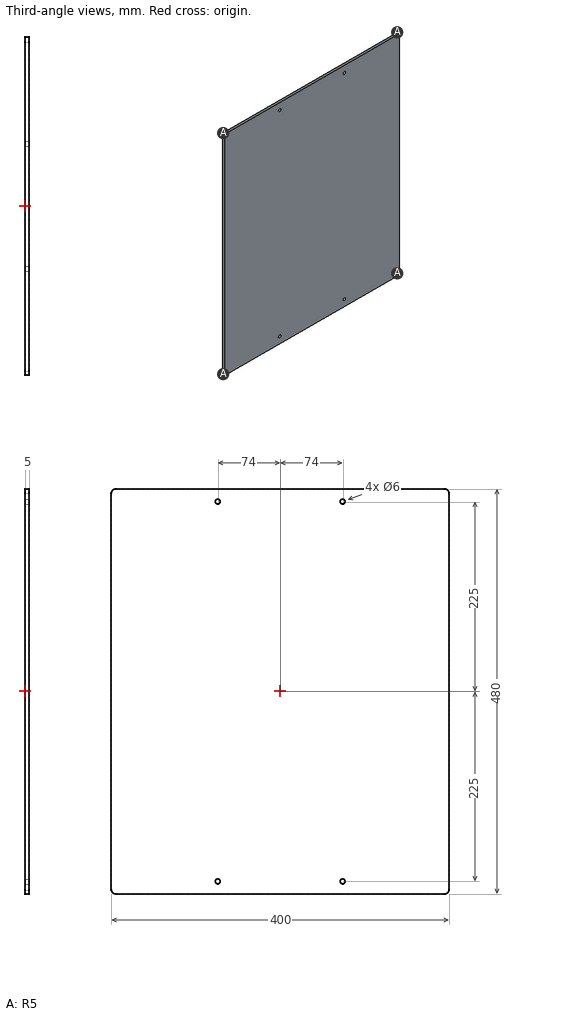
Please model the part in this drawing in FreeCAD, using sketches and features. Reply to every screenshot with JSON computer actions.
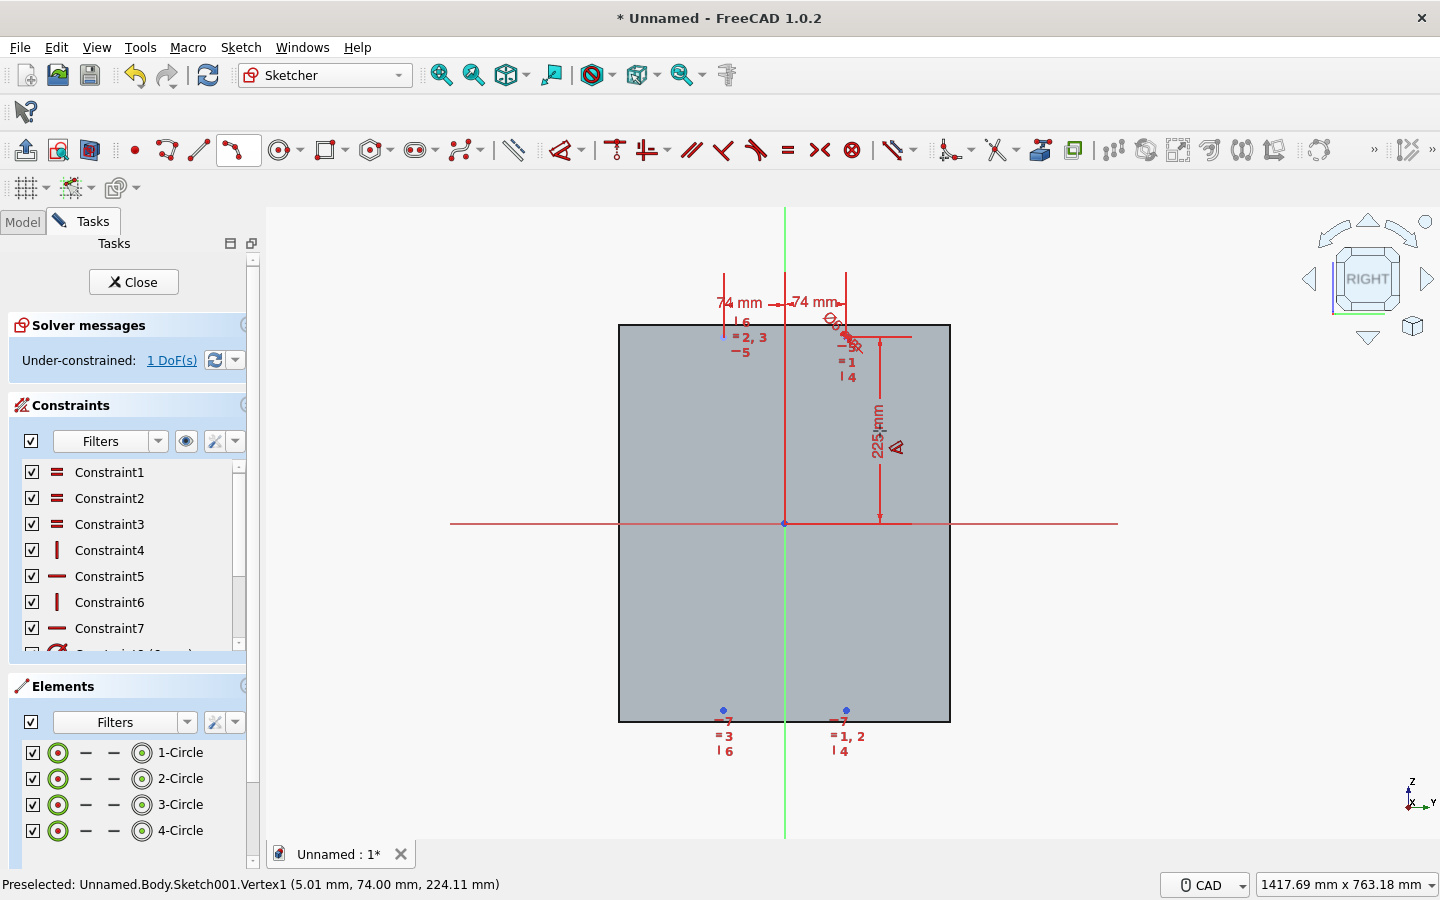
{"action": "left_click", "coordinate": [846, 711]}
{"action": "left_click", "coordinate": [880, 617]}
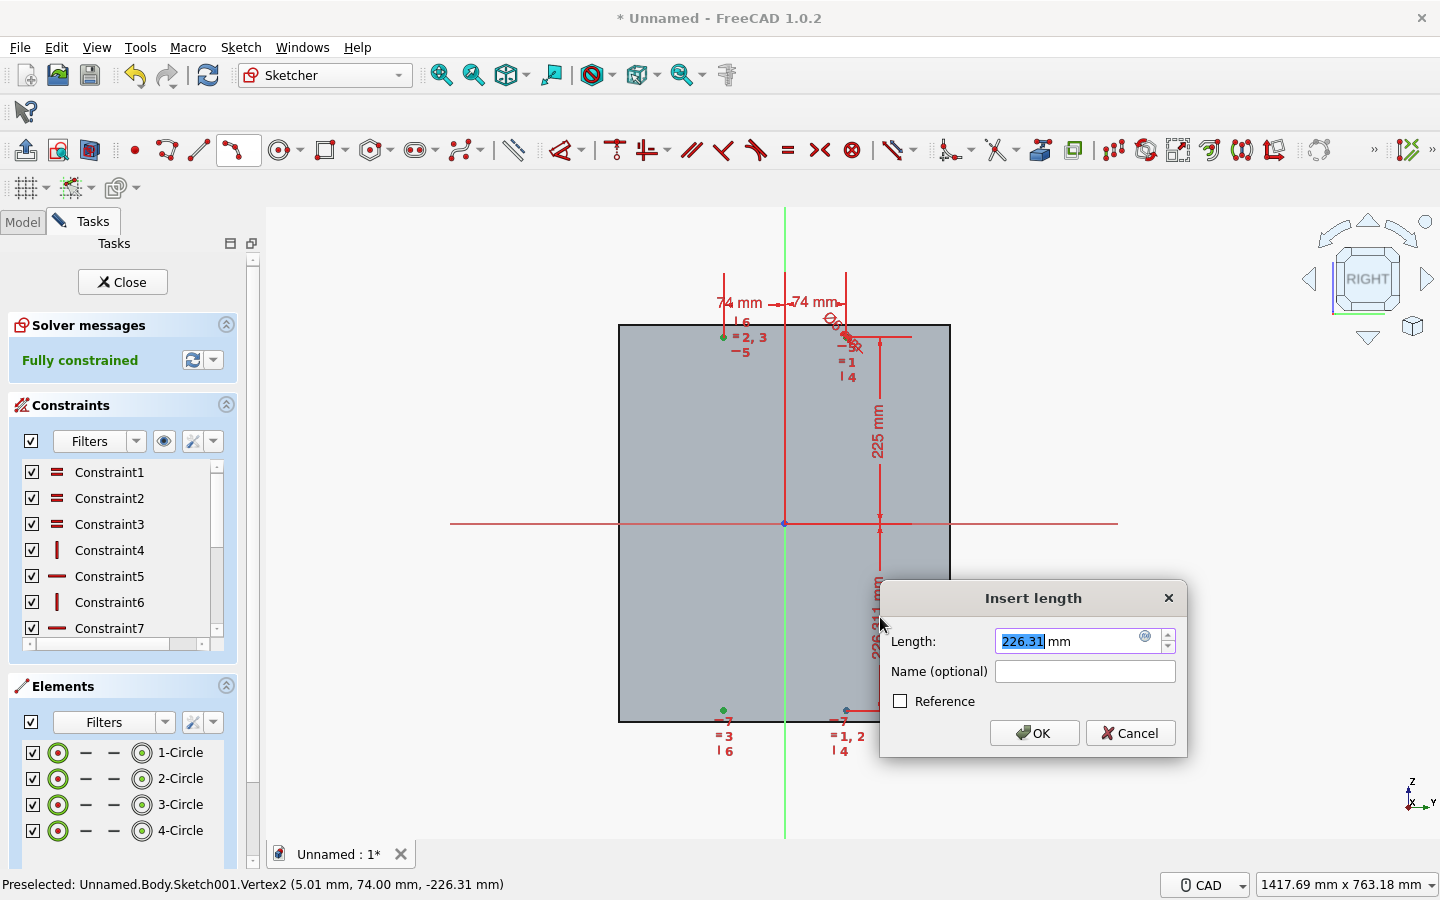
{"action": "type", "text": "225"}
{"action": "key", "text": "Return"}
{"action": "key", "text": "Escape"}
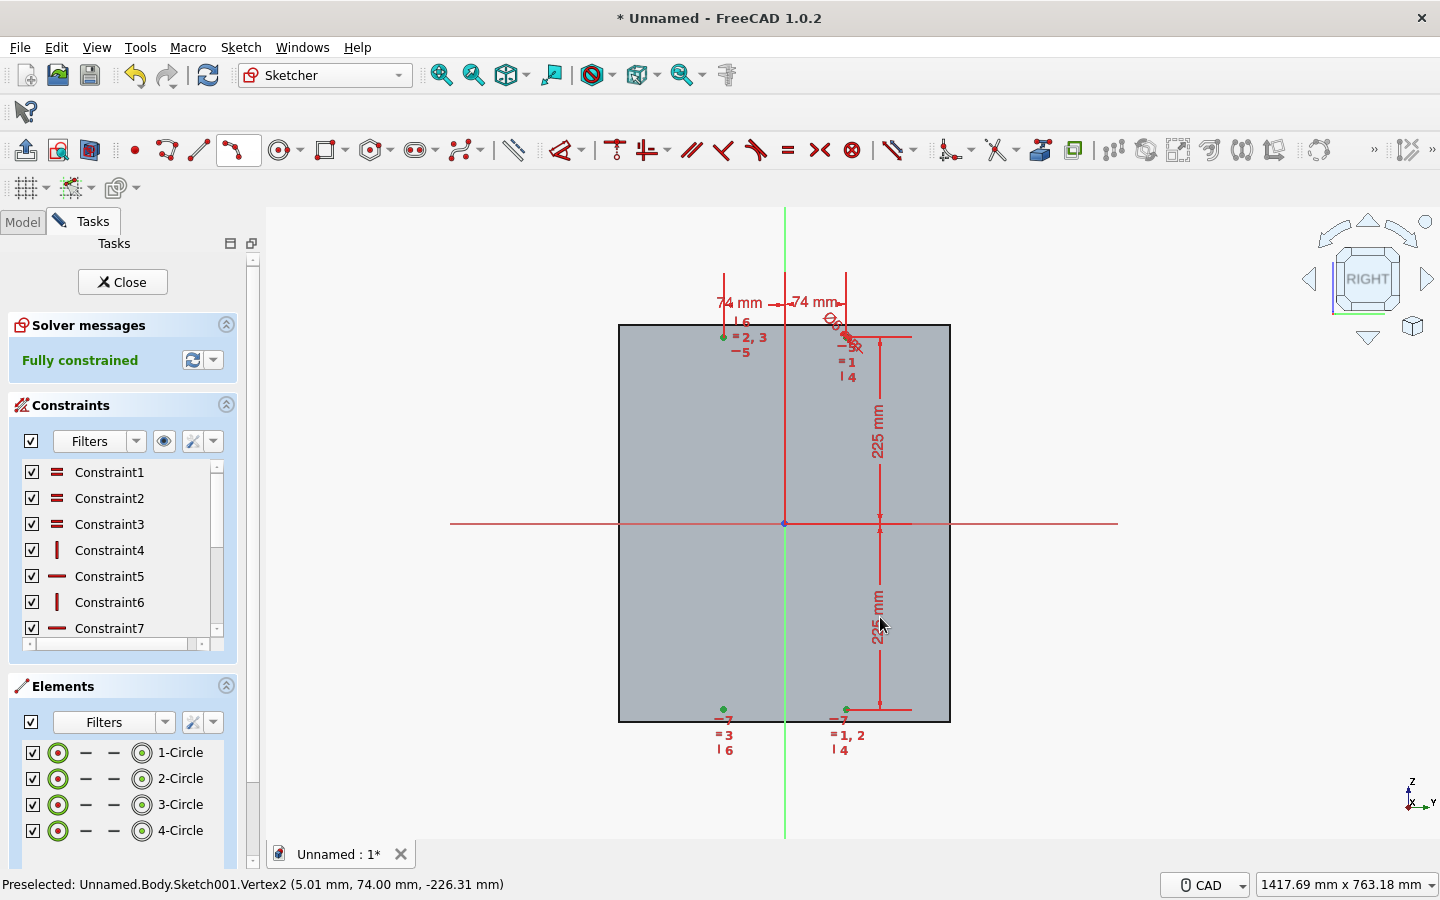
{"action": "left_click", "coordinate": [123, 282]}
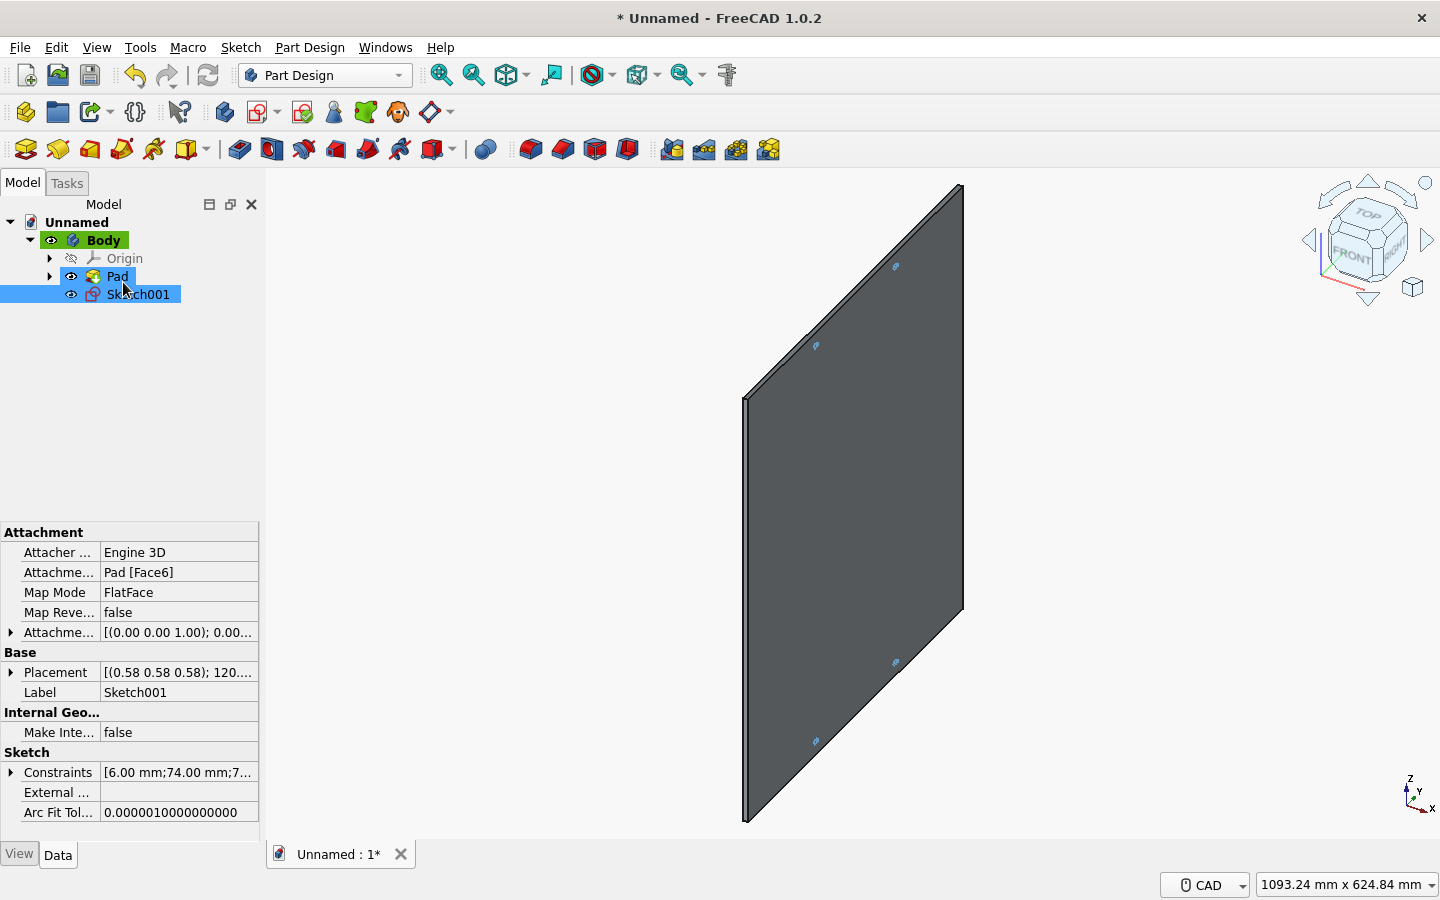
{"action": "left_click", "coordinate": [240, 150]}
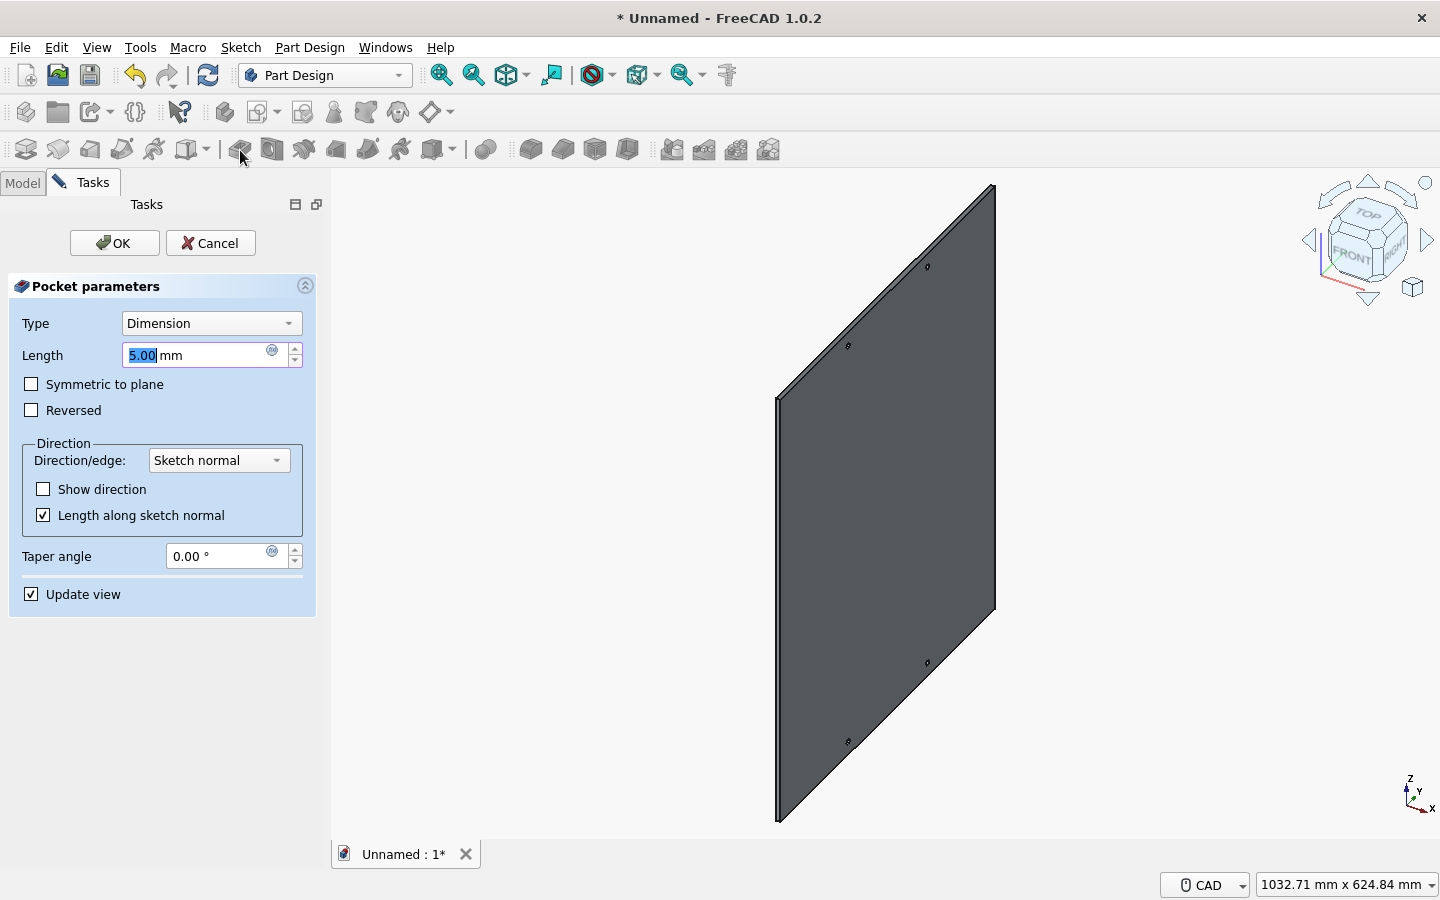
{"action": "left_click", "coordinate": [212, 324]}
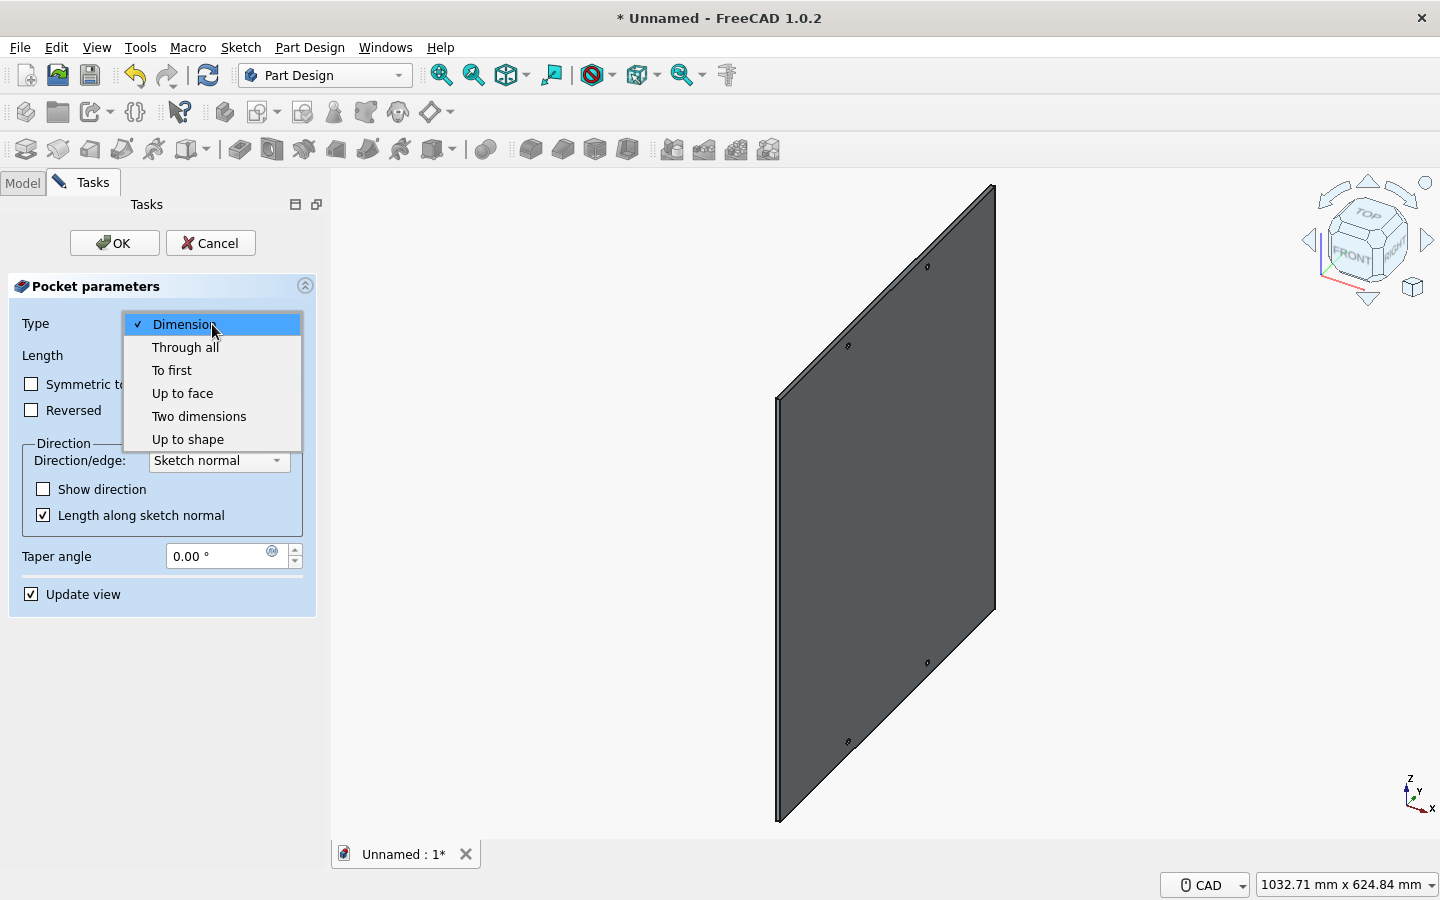
{"action": "left_click", "coordinate": [212, 348]}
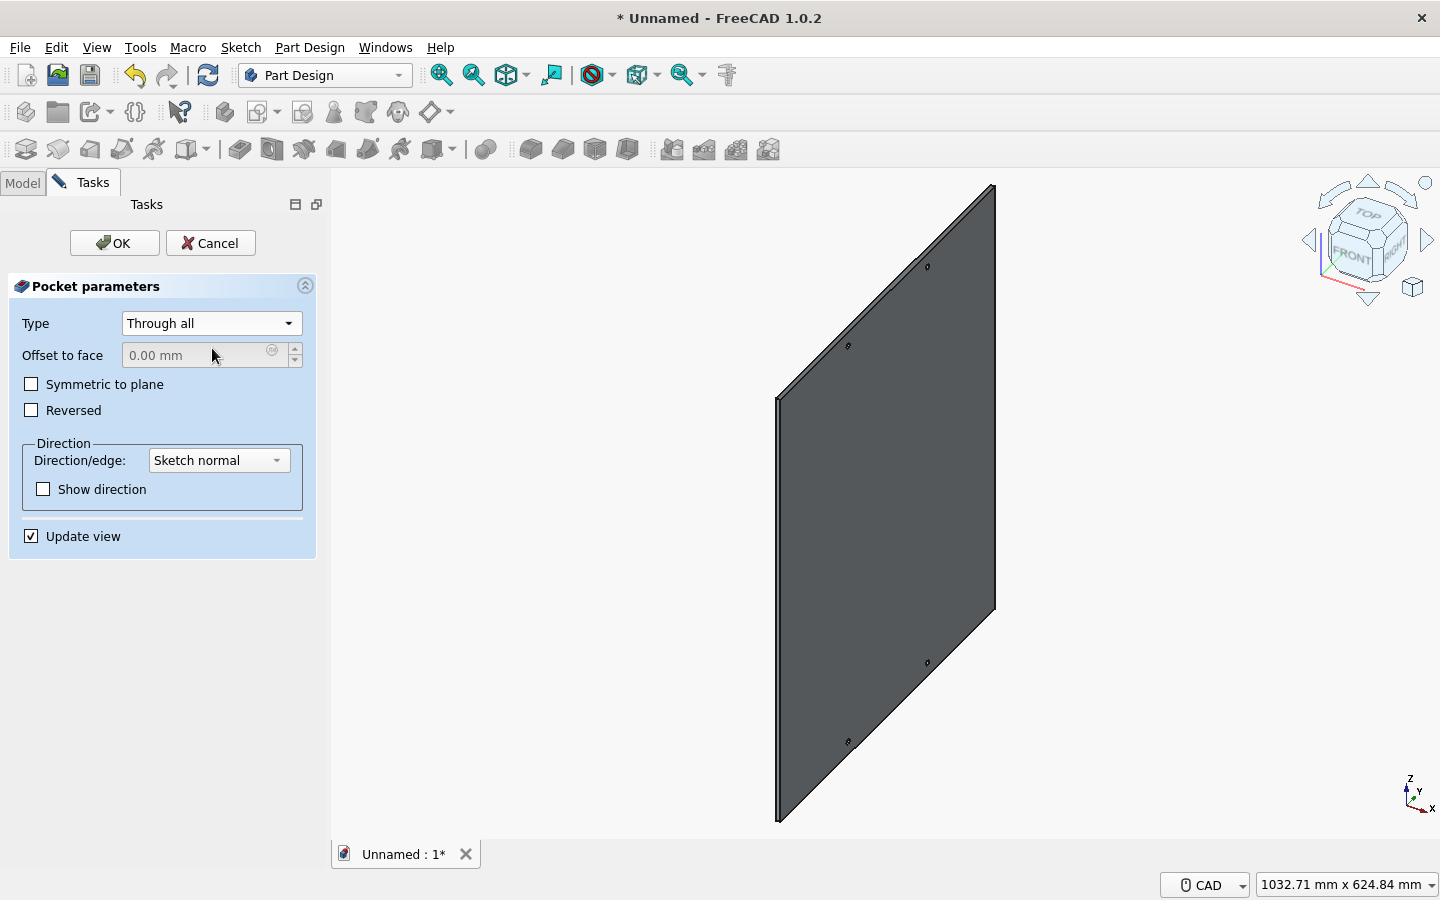
{"action": "left_click", "coordinate": [115, 243]}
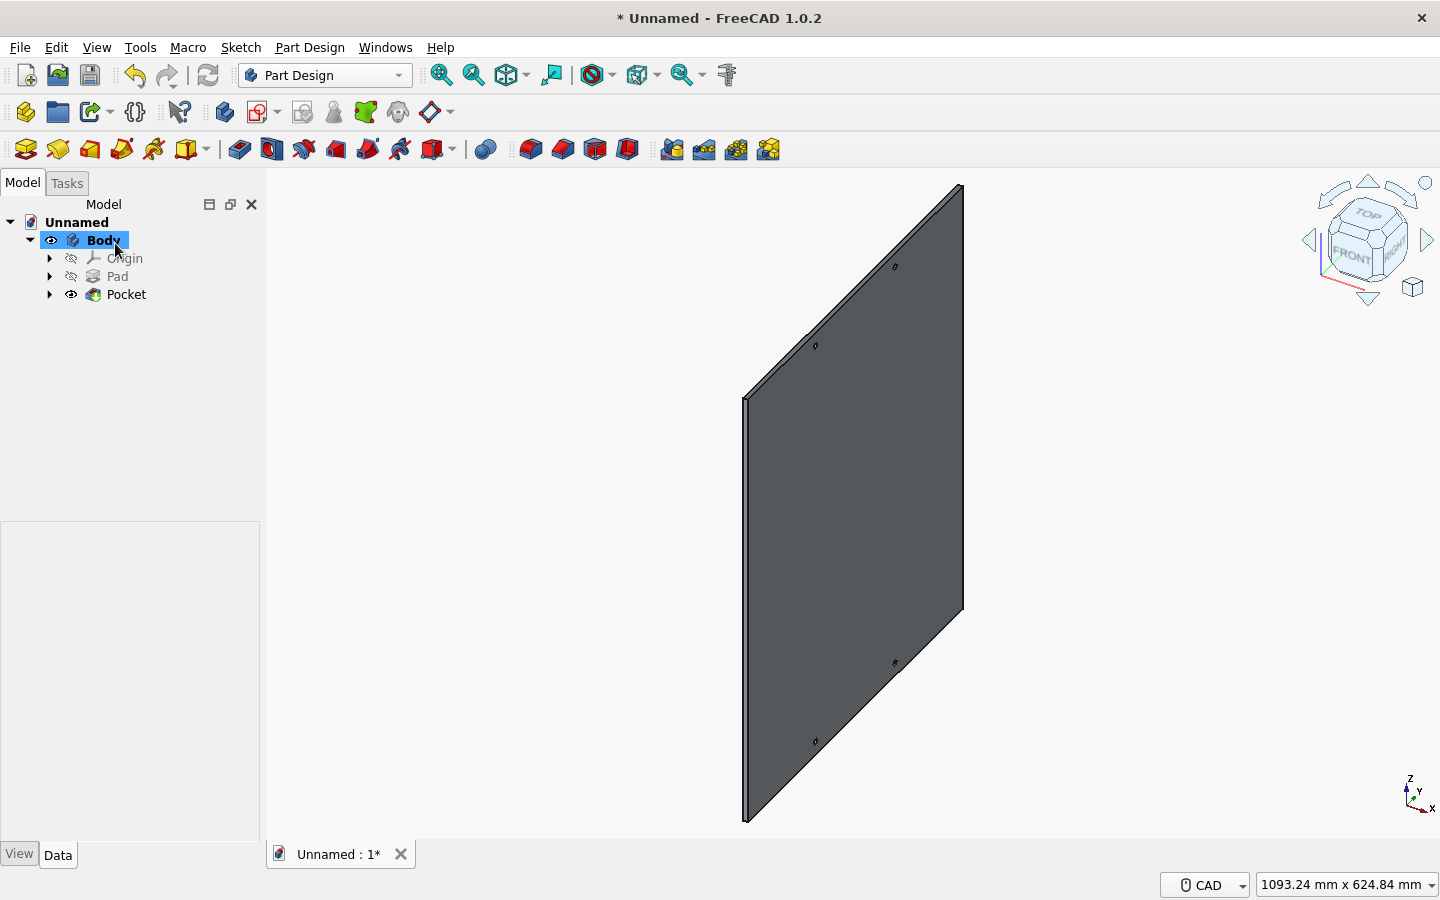
{"action": "key", "text": "0"}